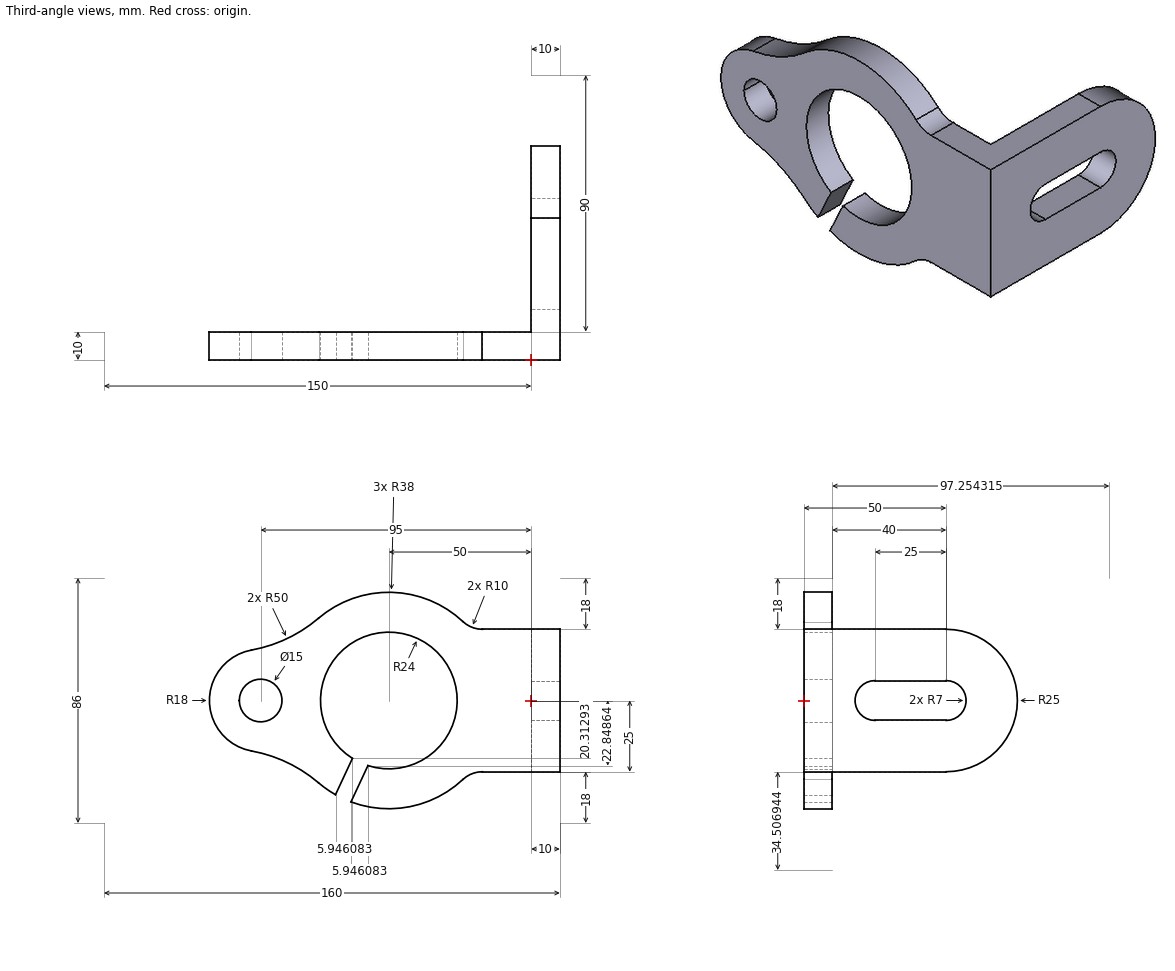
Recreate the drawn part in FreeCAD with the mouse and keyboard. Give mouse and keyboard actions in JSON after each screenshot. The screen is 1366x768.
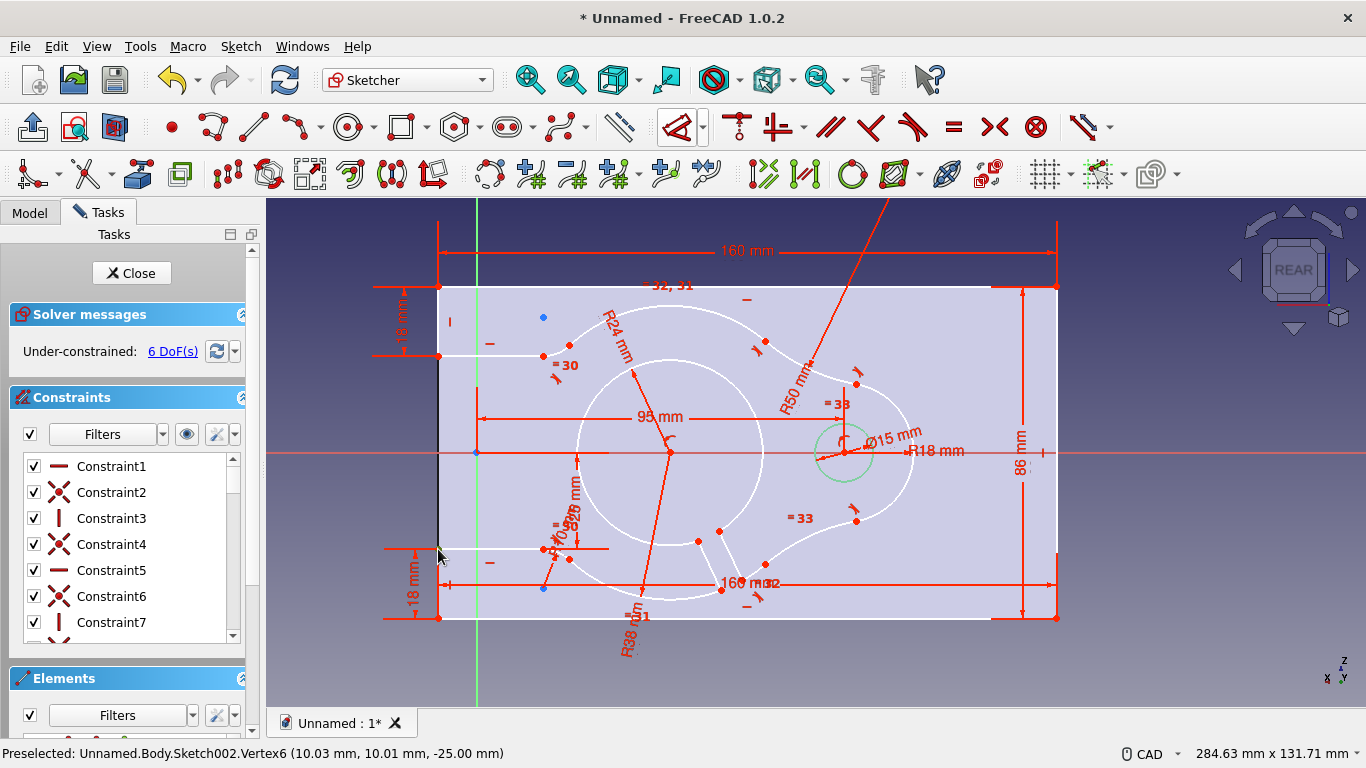
{"action": "key", "text": "l"}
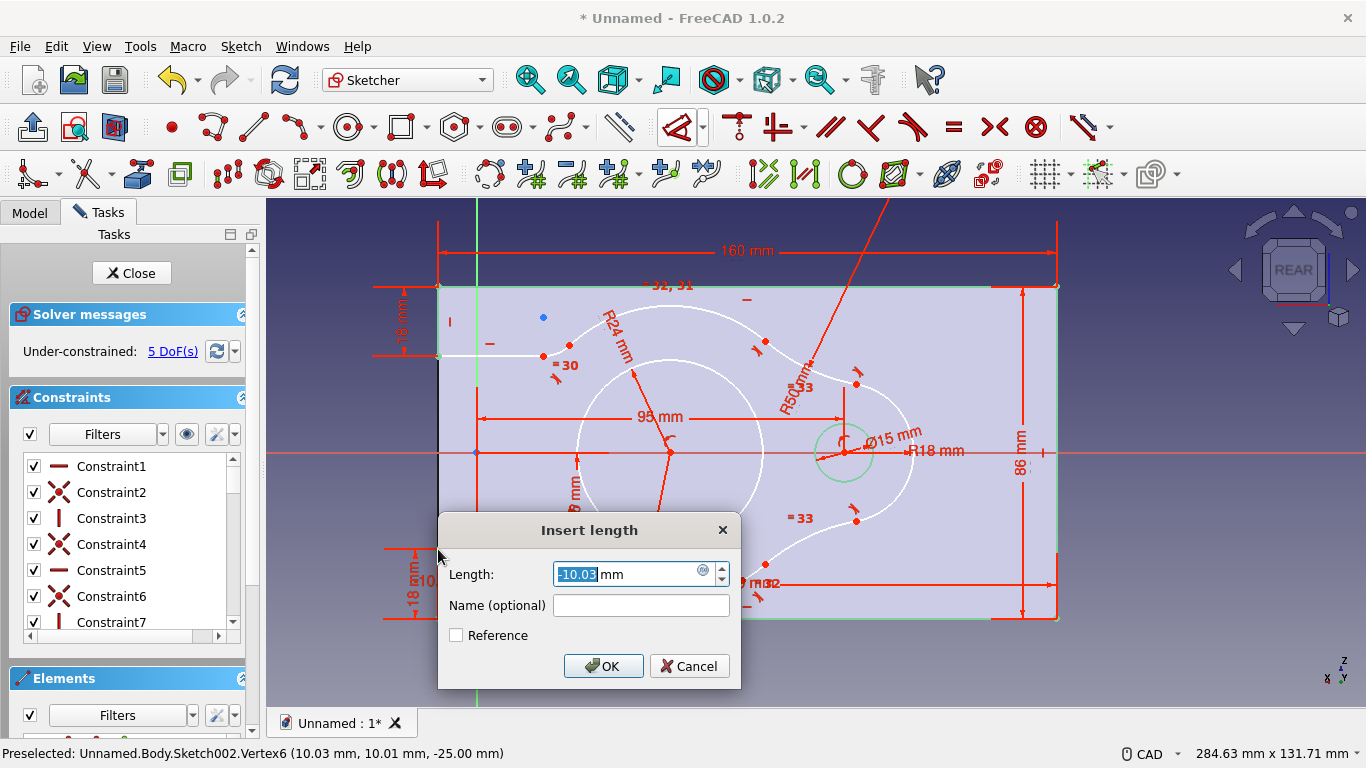
{"action": "type", "text": "-10"}
{"action": "key", "text": "Return"}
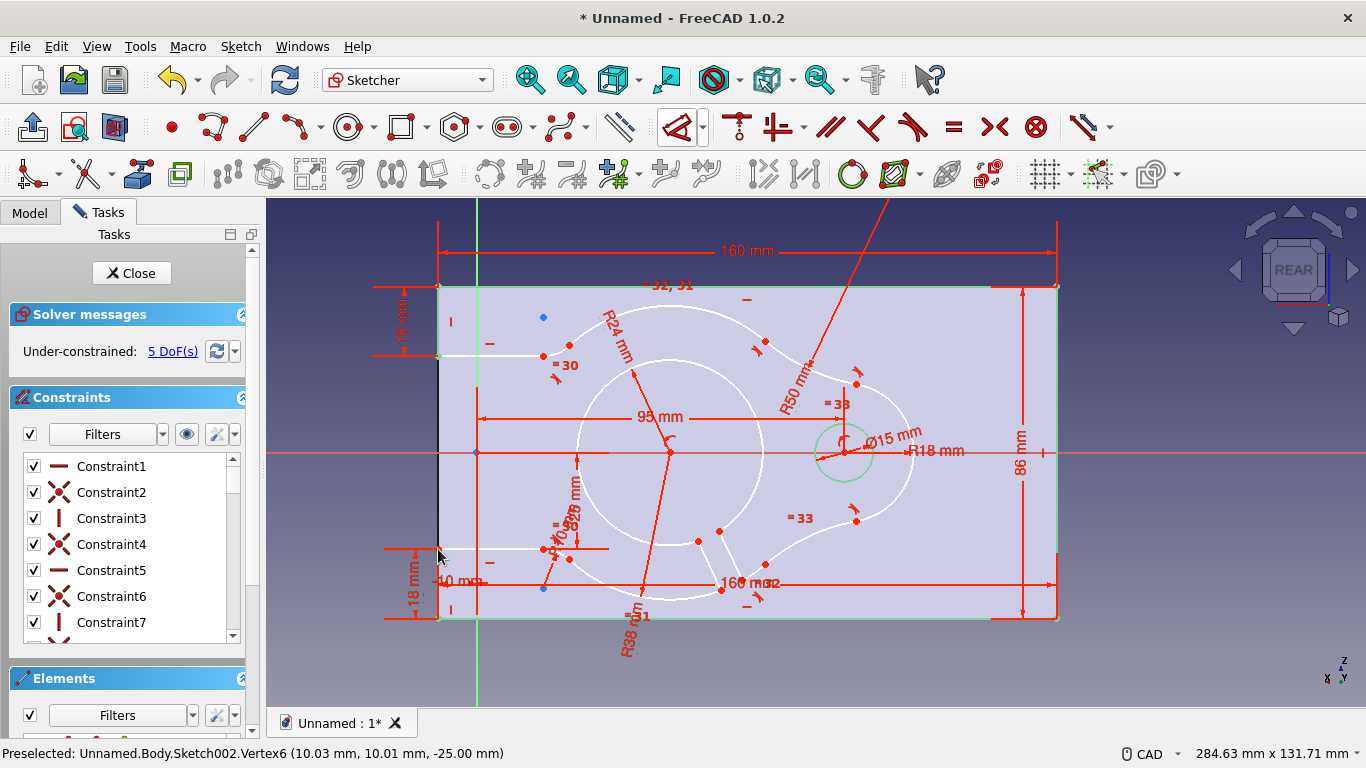
{"action": "left_click", "coordinate": [670, 453]}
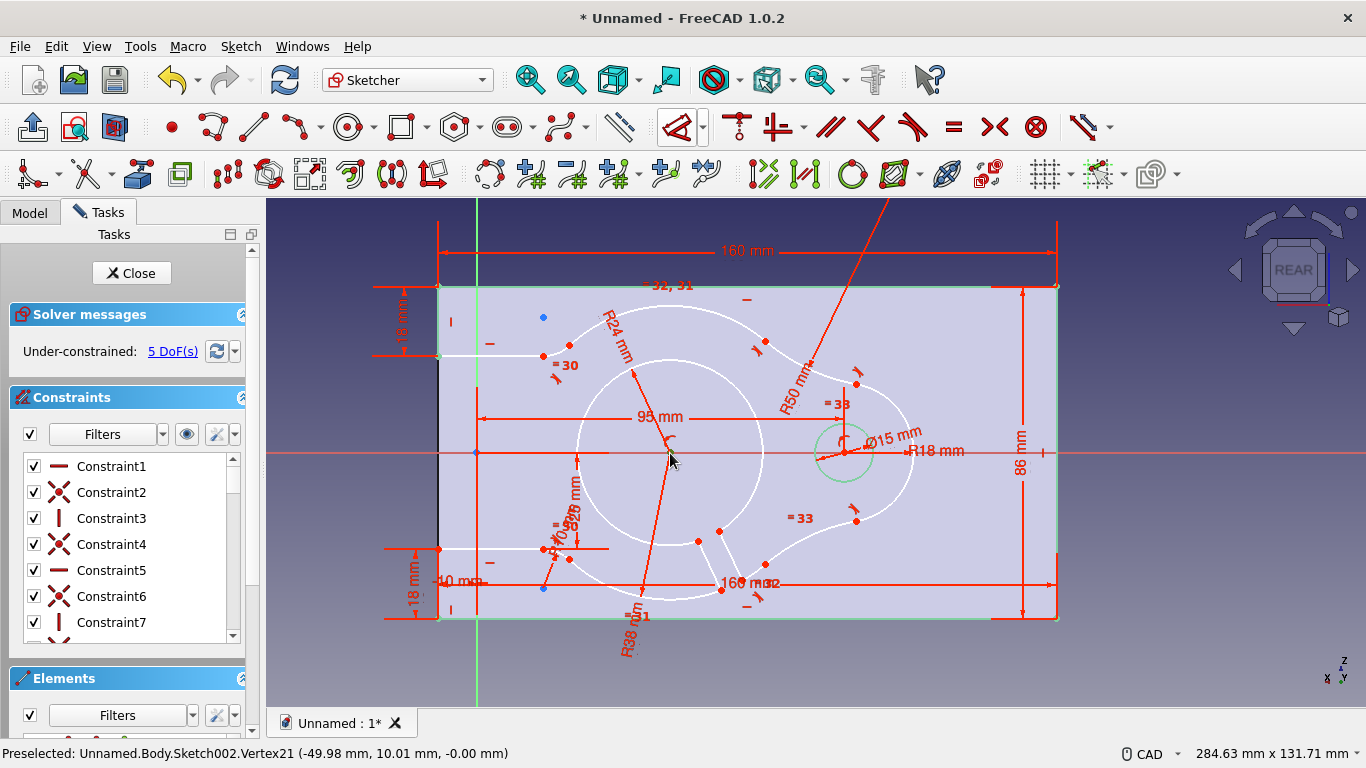
{"action": "key", "text": "l"}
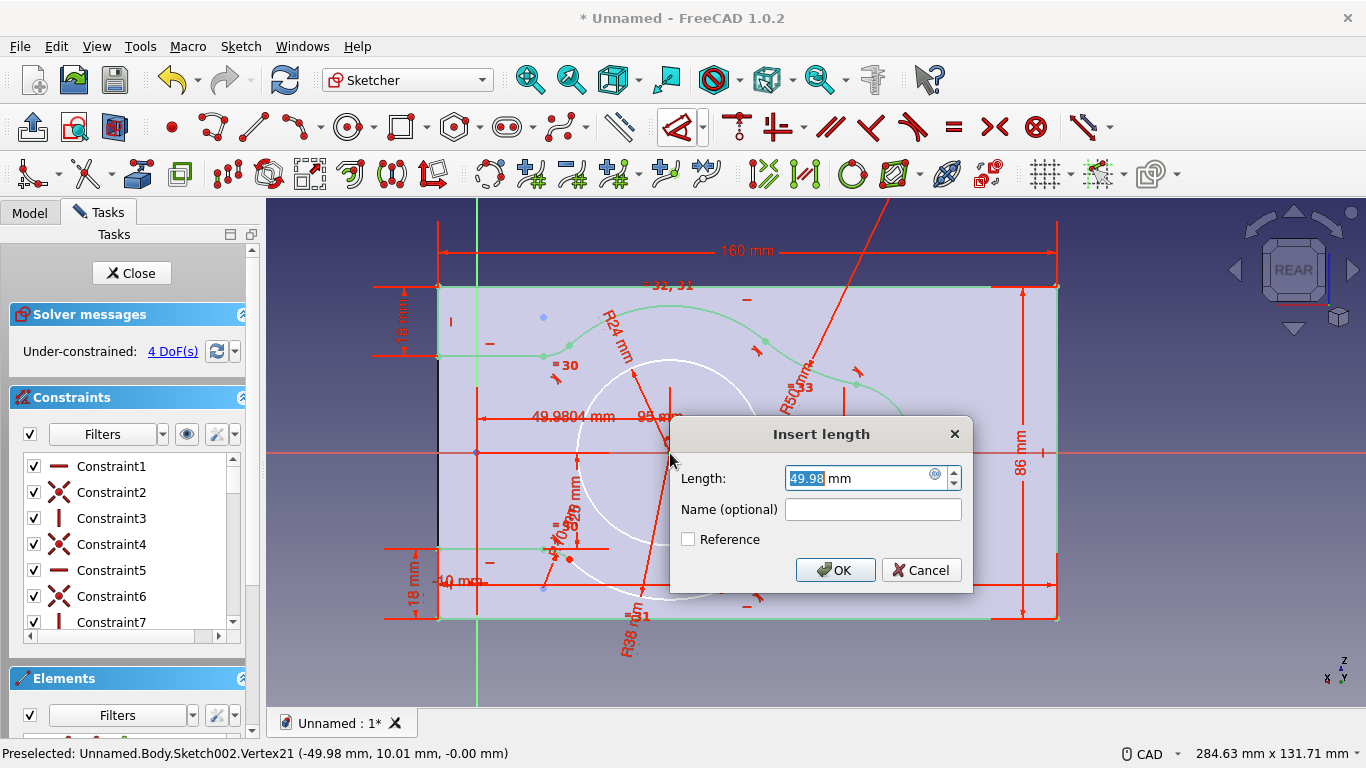
{"action": "type", "text": "50"}
{"action": "key", "text": "Return"}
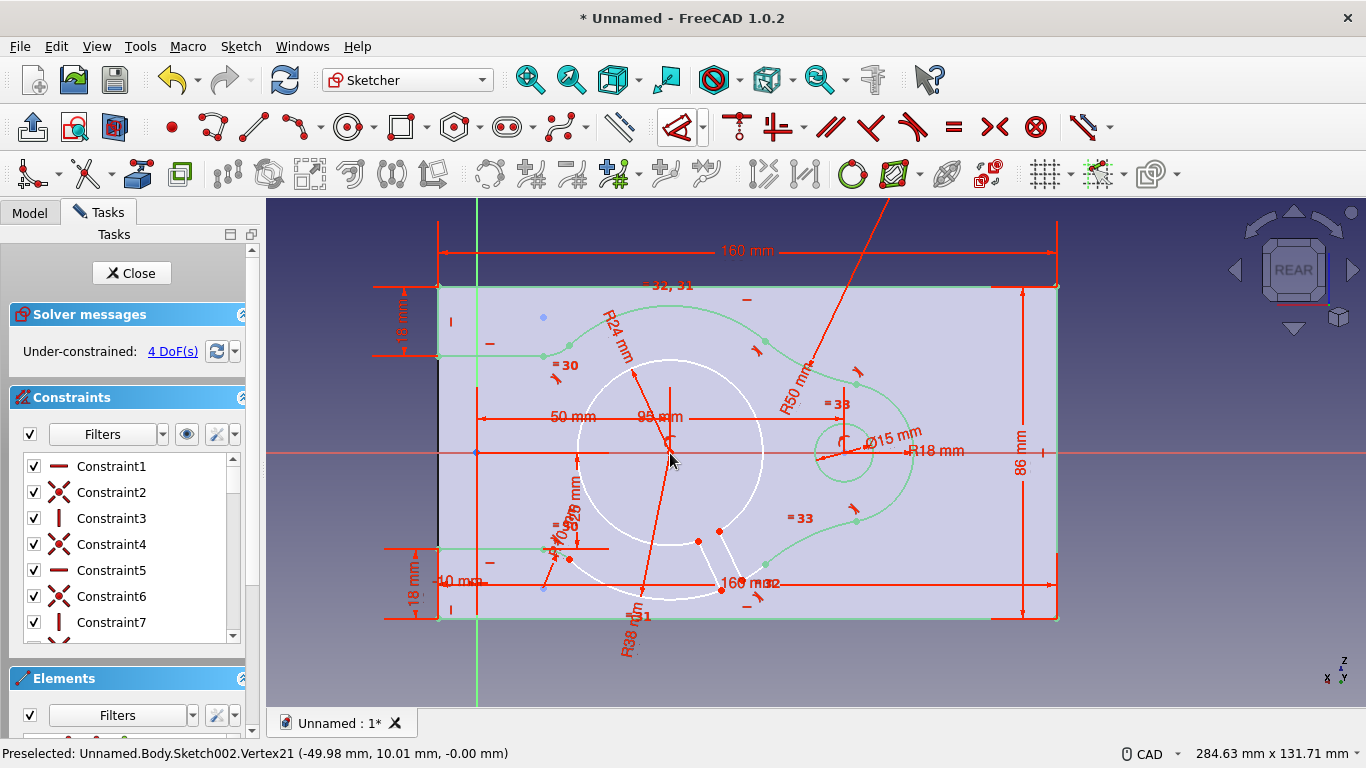
{"action": "left_click", "coordinate": [719, 532]}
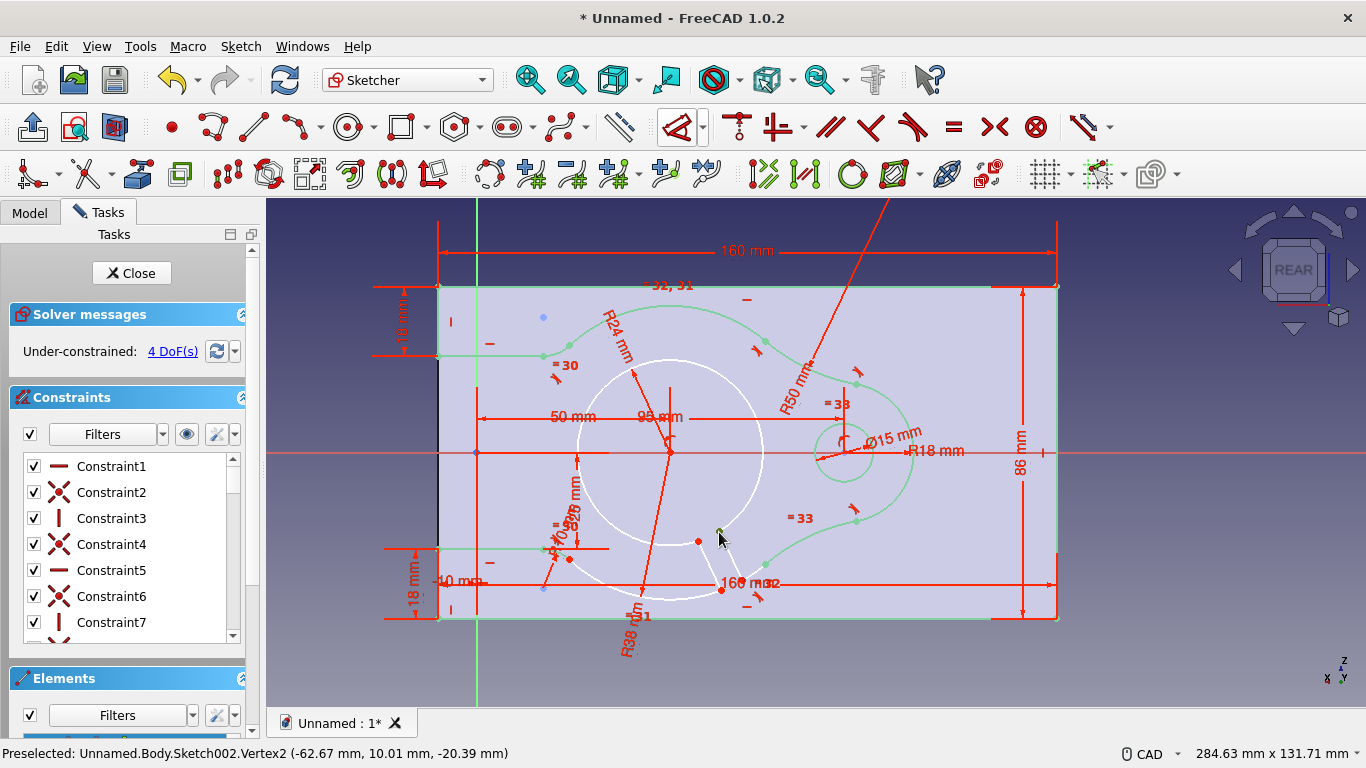
{"action": "left_click", "coordinate": [702, 128]}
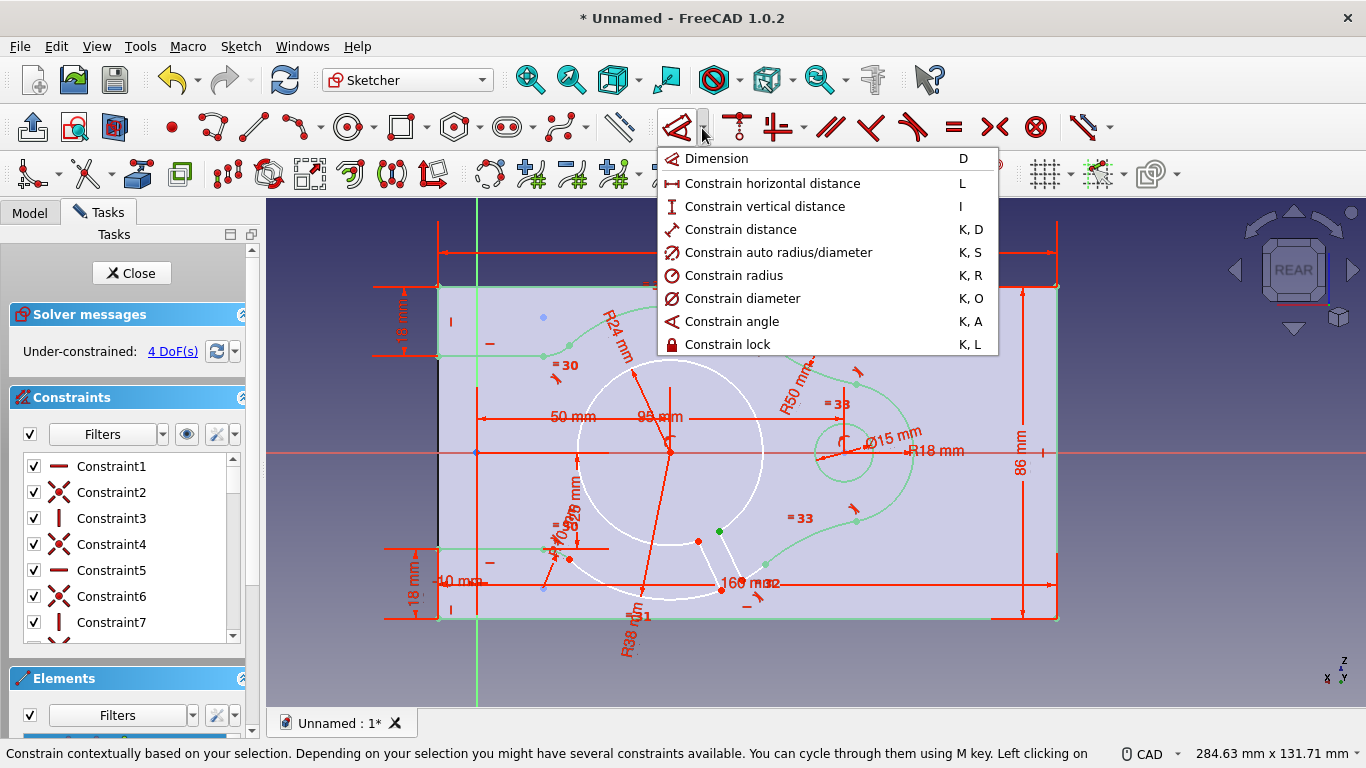
{"action": "left_click", "coordinate": [828, 206]}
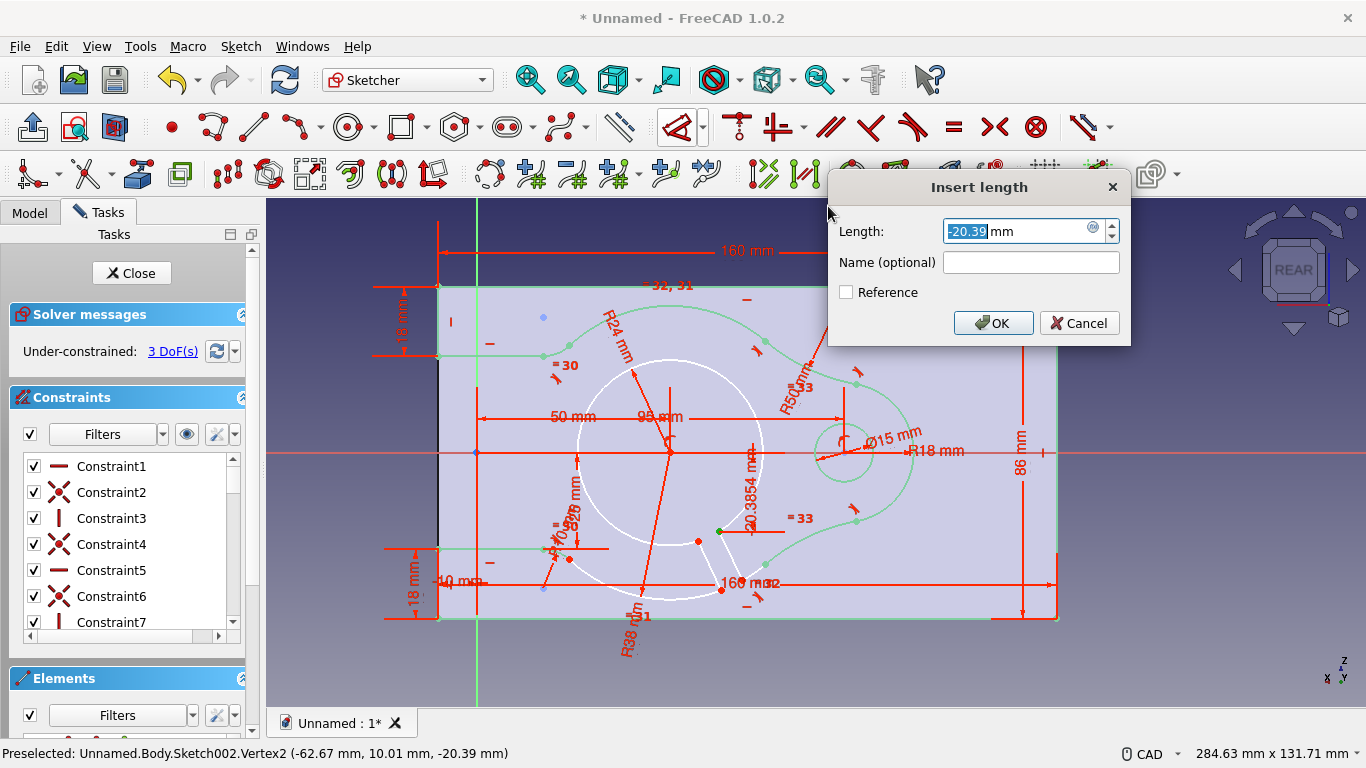
{"action": "type", "text": "-20.31293"}
{"action": "key", "text": "Return"}